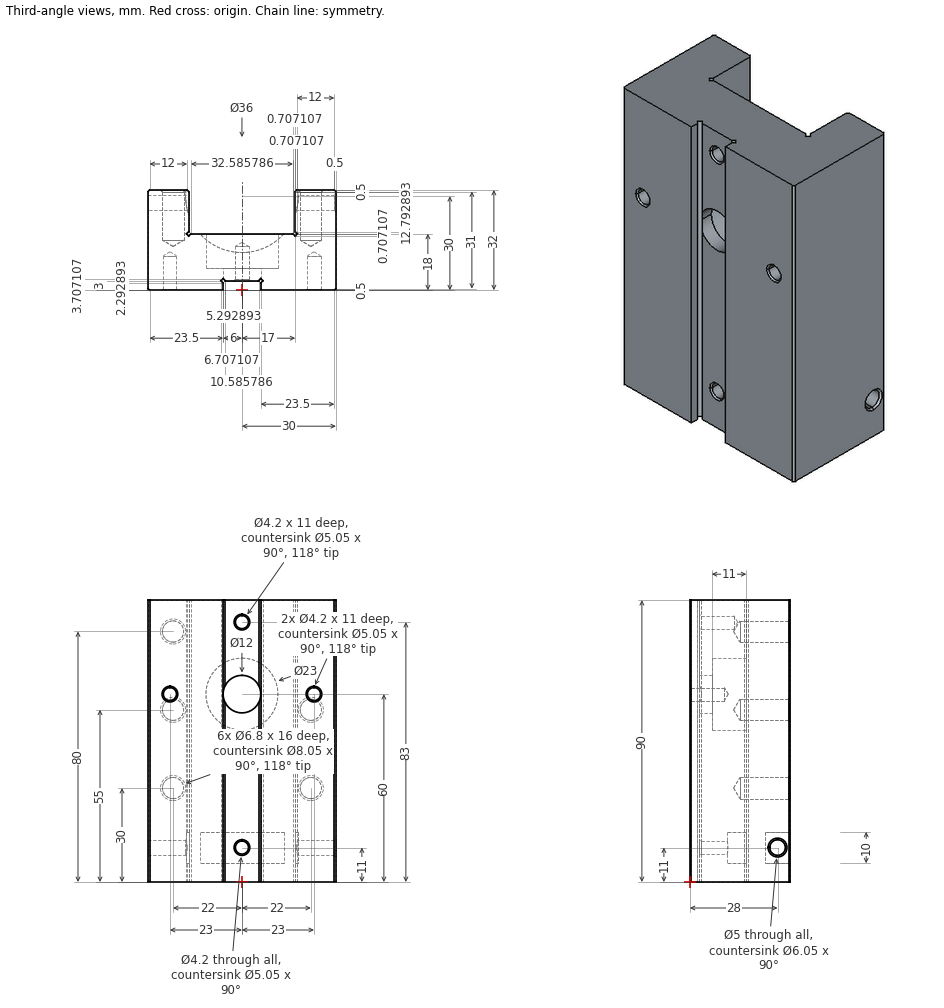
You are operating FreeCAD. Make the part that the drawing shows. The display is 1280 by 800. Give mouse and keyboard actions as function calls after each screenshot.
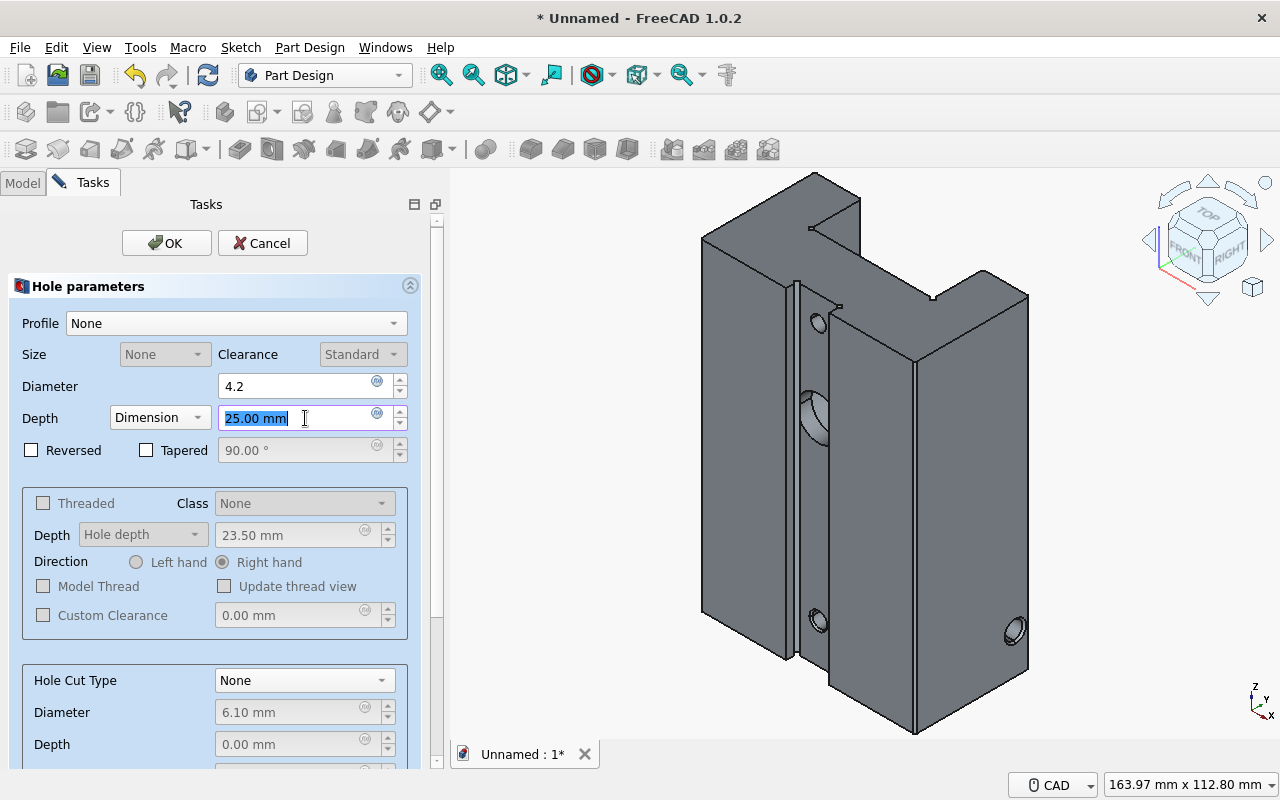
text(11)
key(Tab)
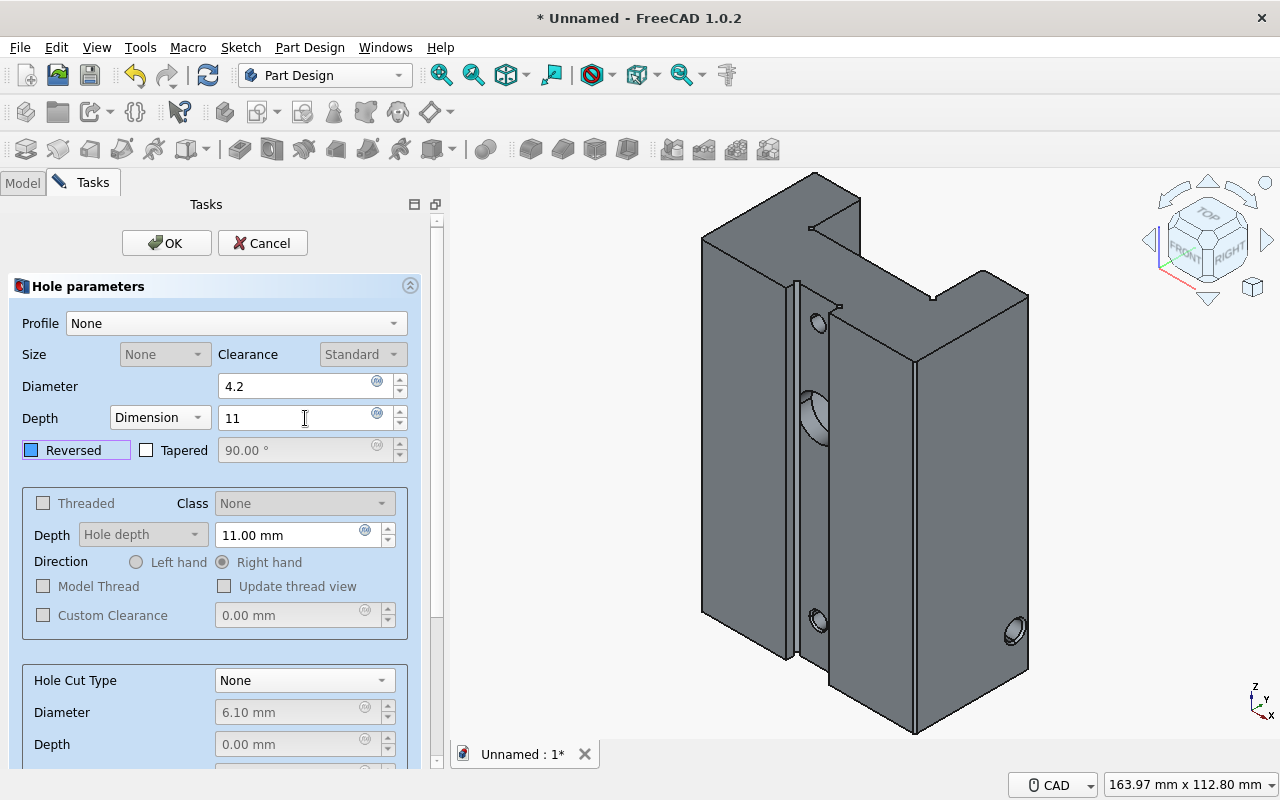
click(306, 680)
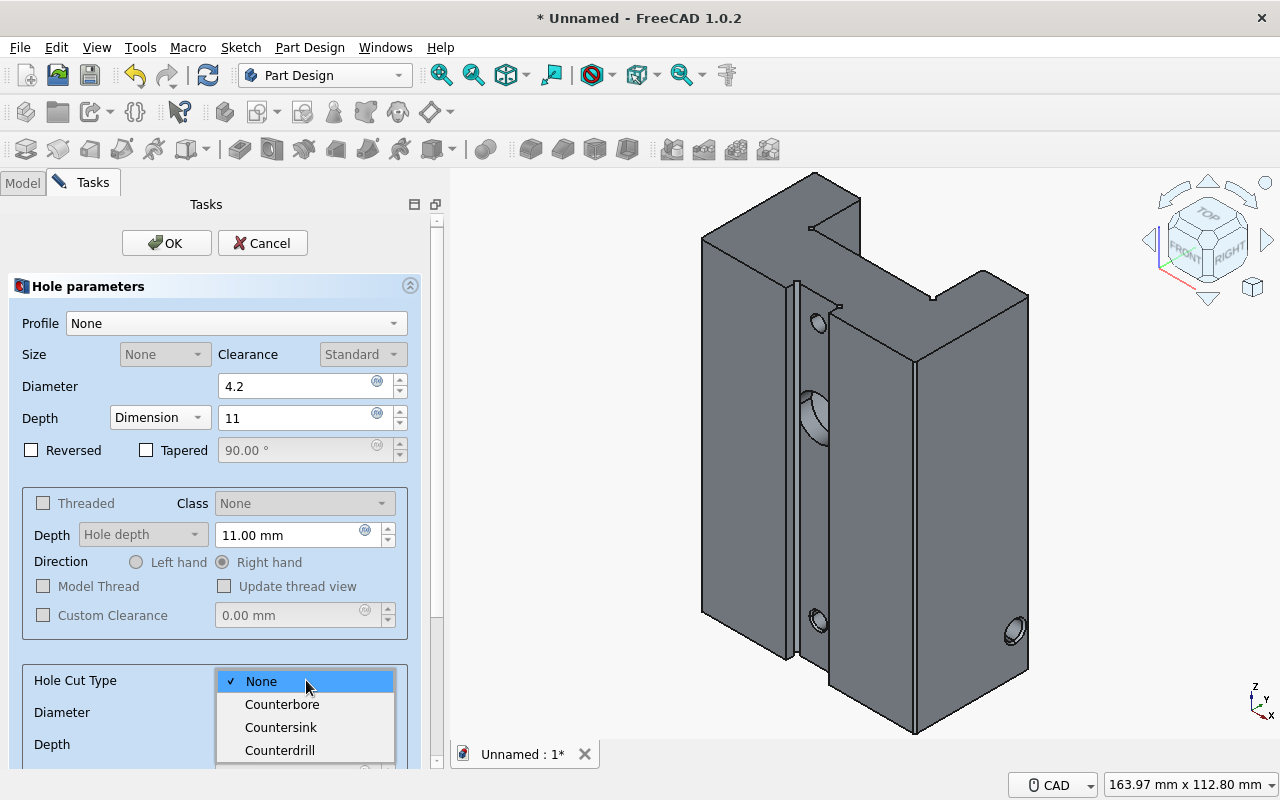
click(304, 728)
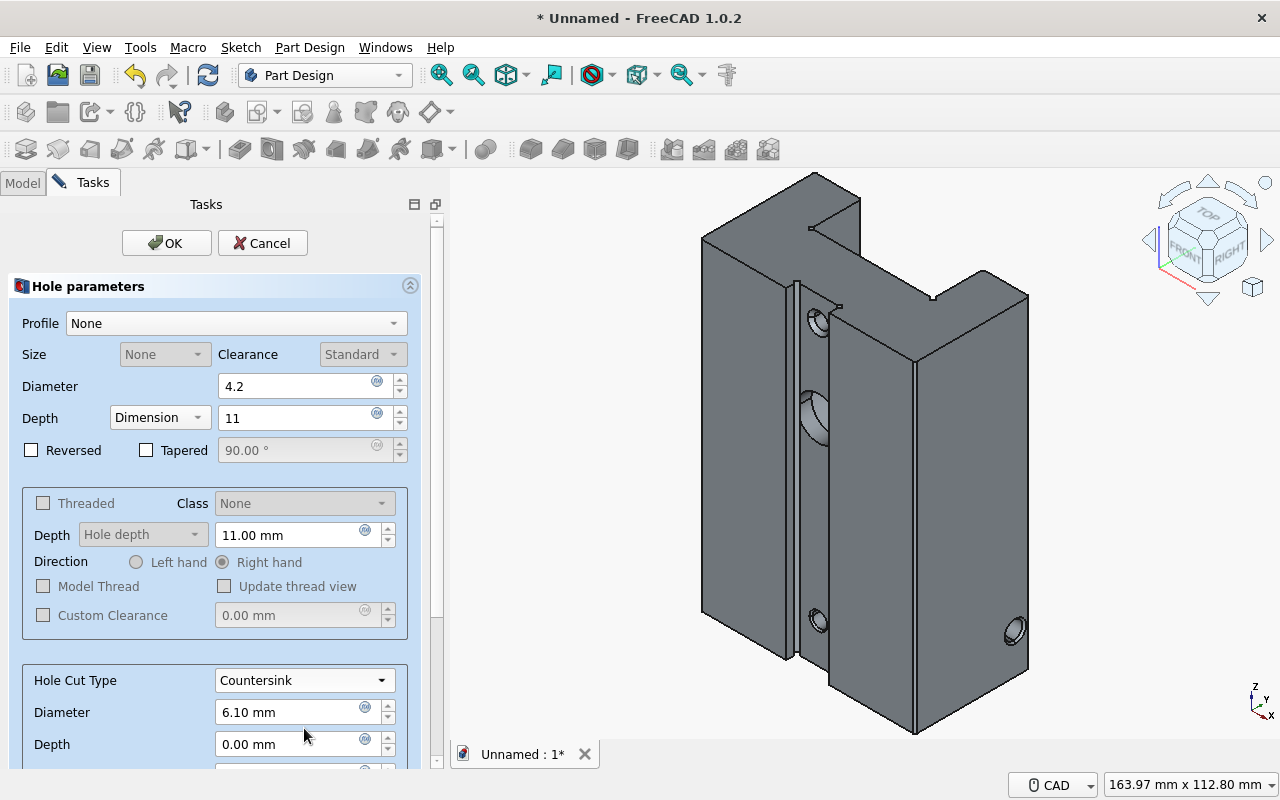
triple_click(298, 712)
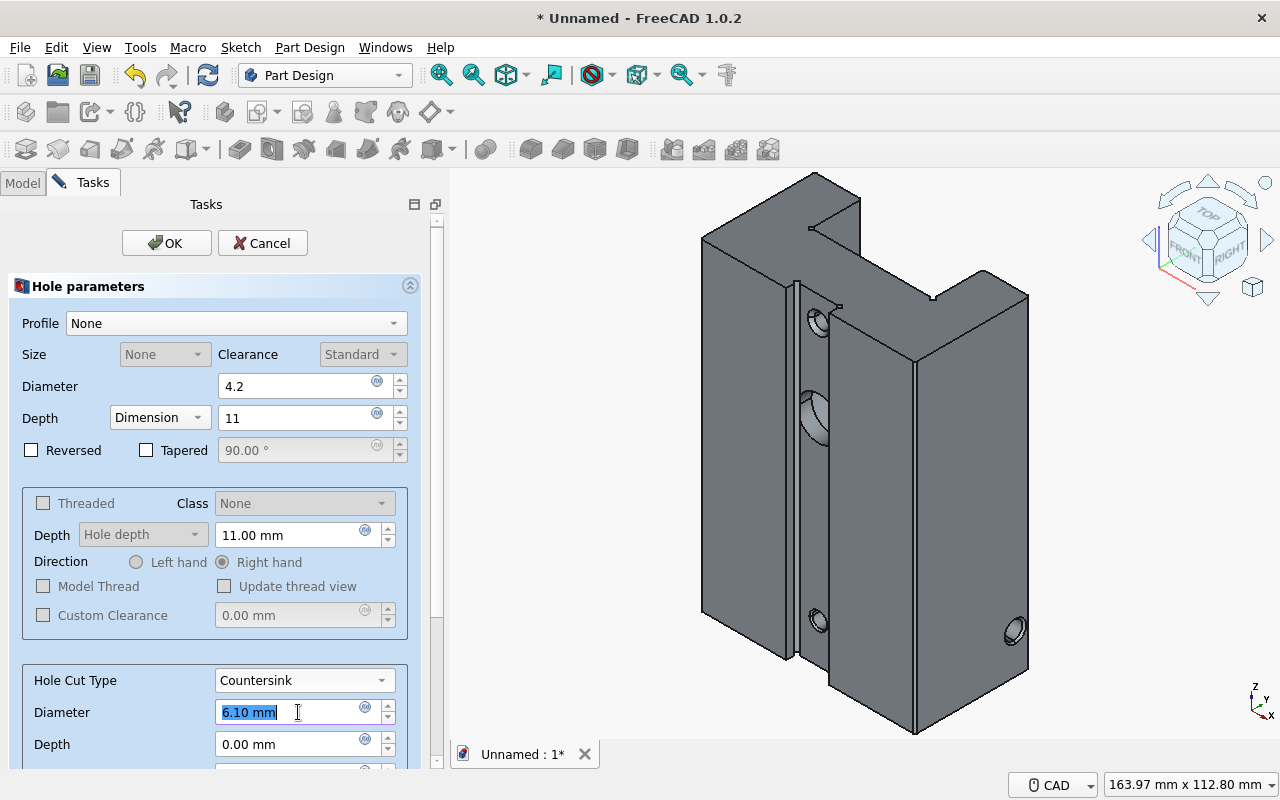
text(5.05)
key(Tab)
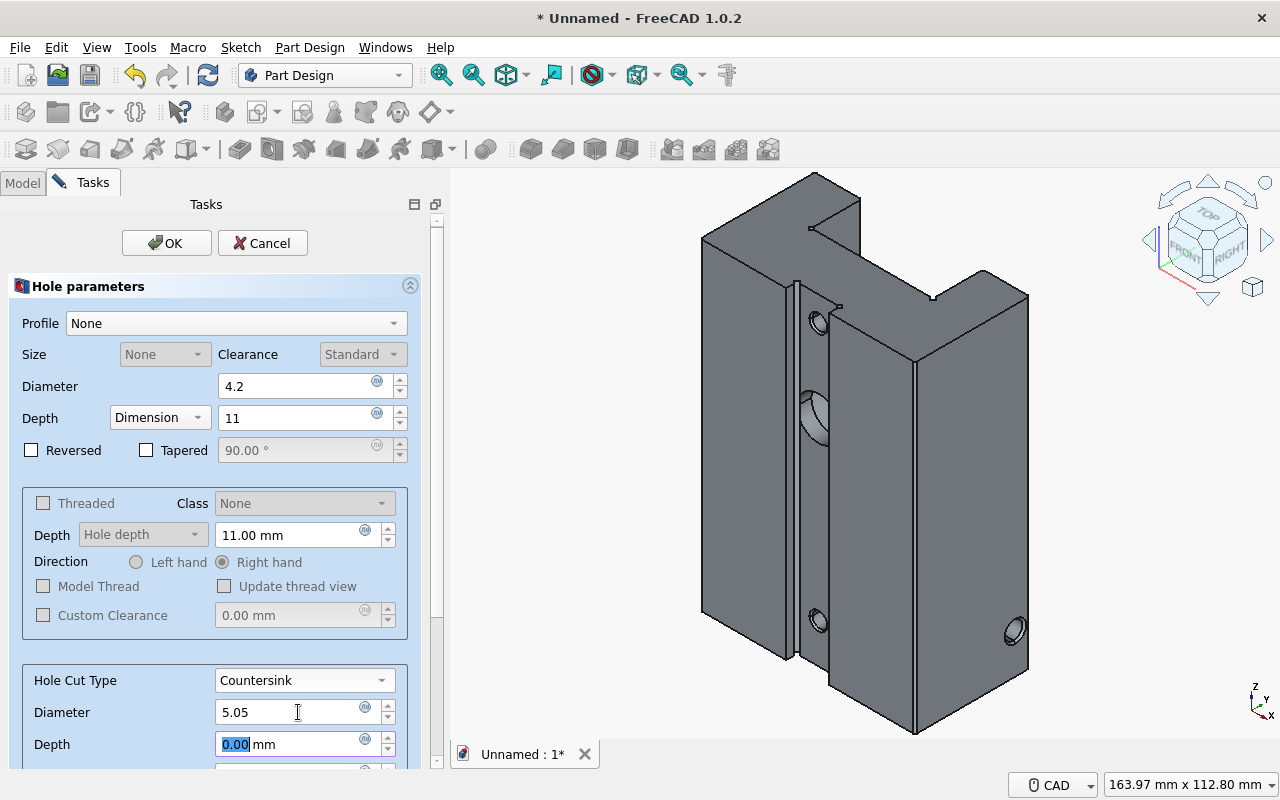
click(167, 243)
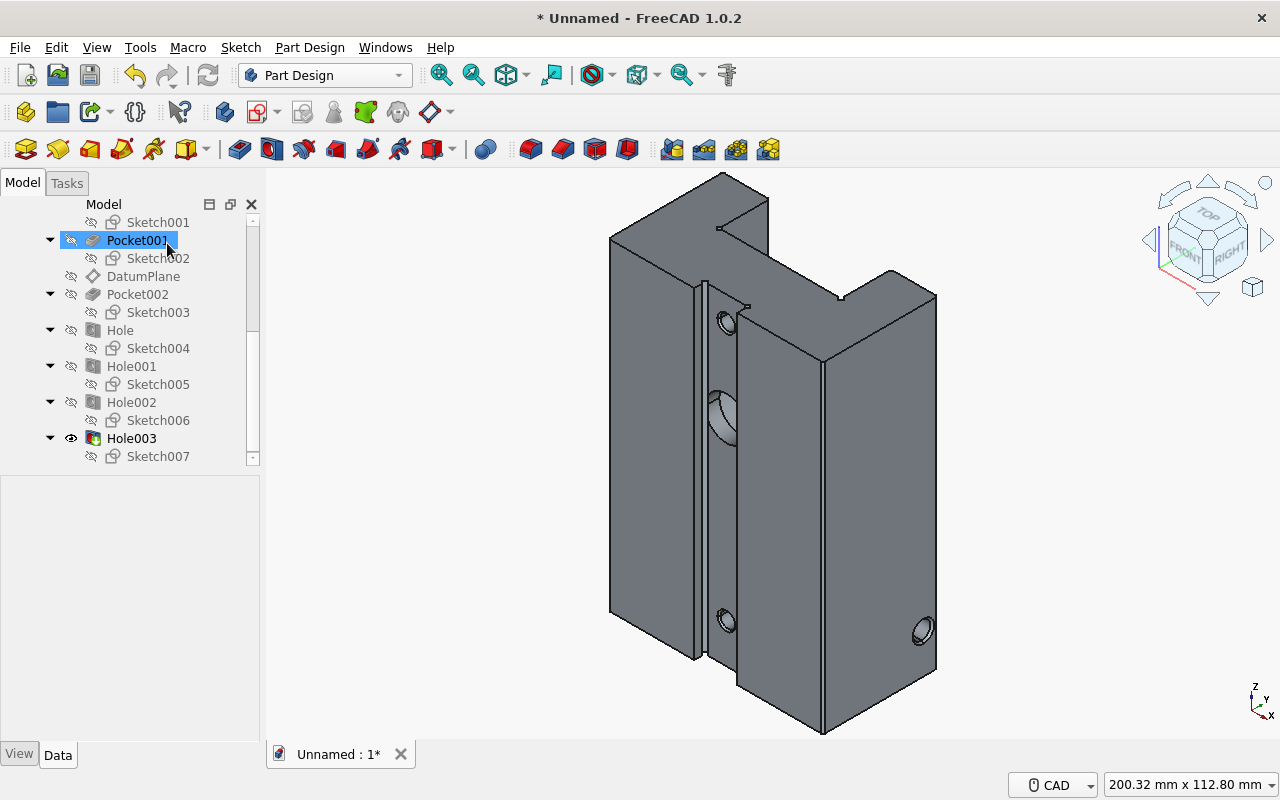
click(258, 112)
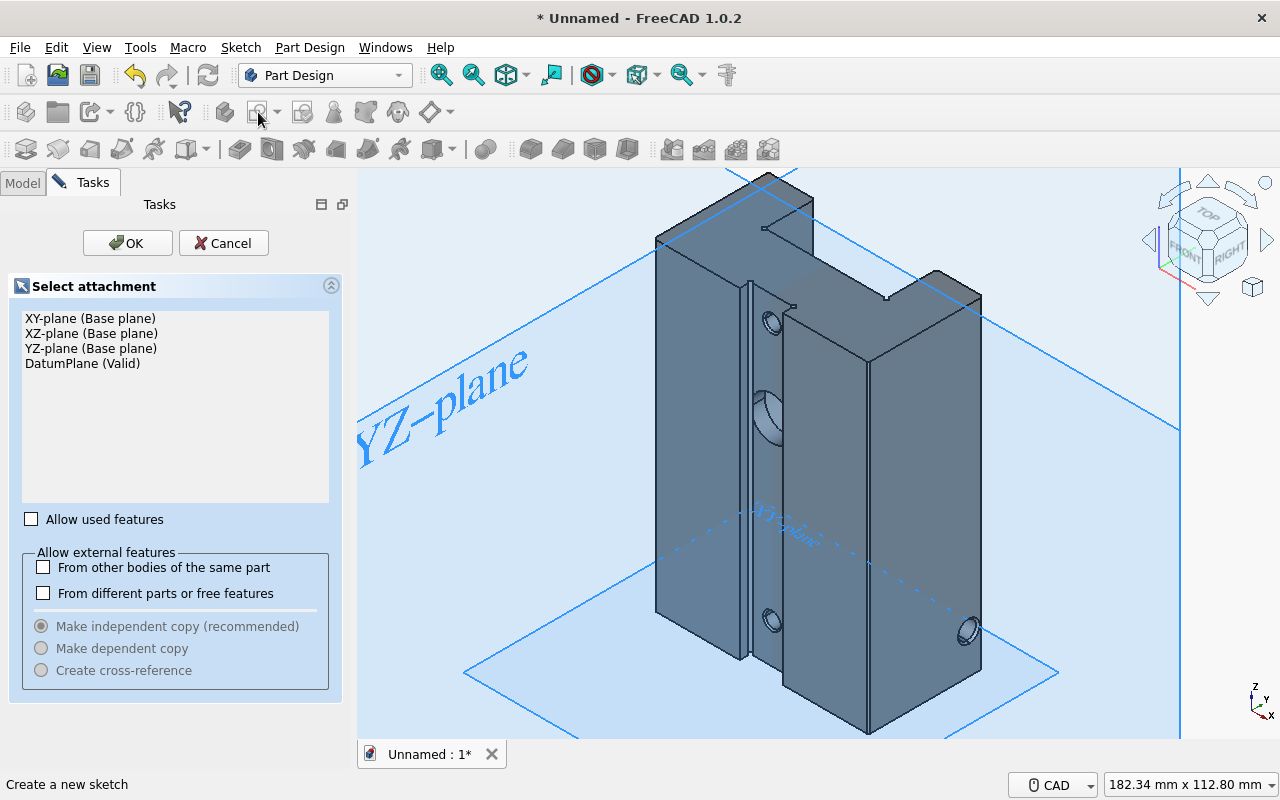
click(82, 334)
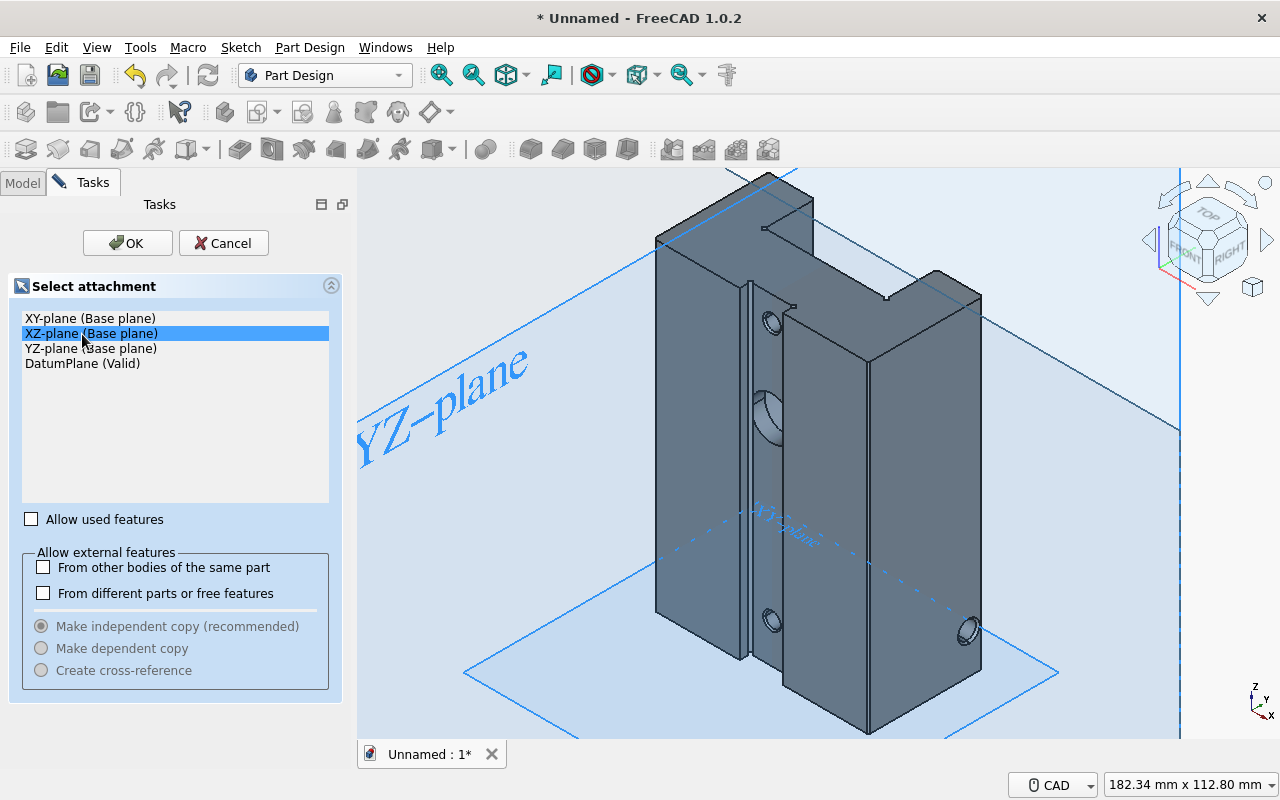
click(128, 243)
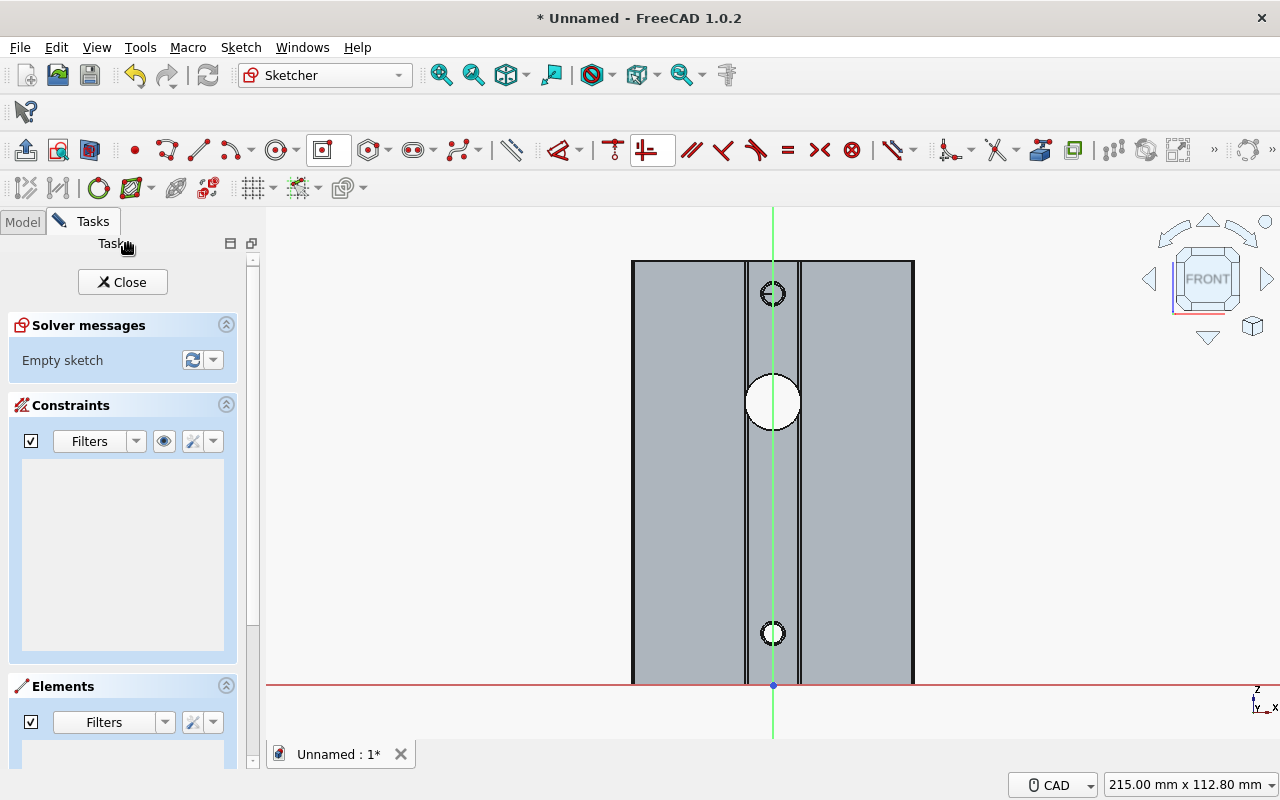
click(276, 150)